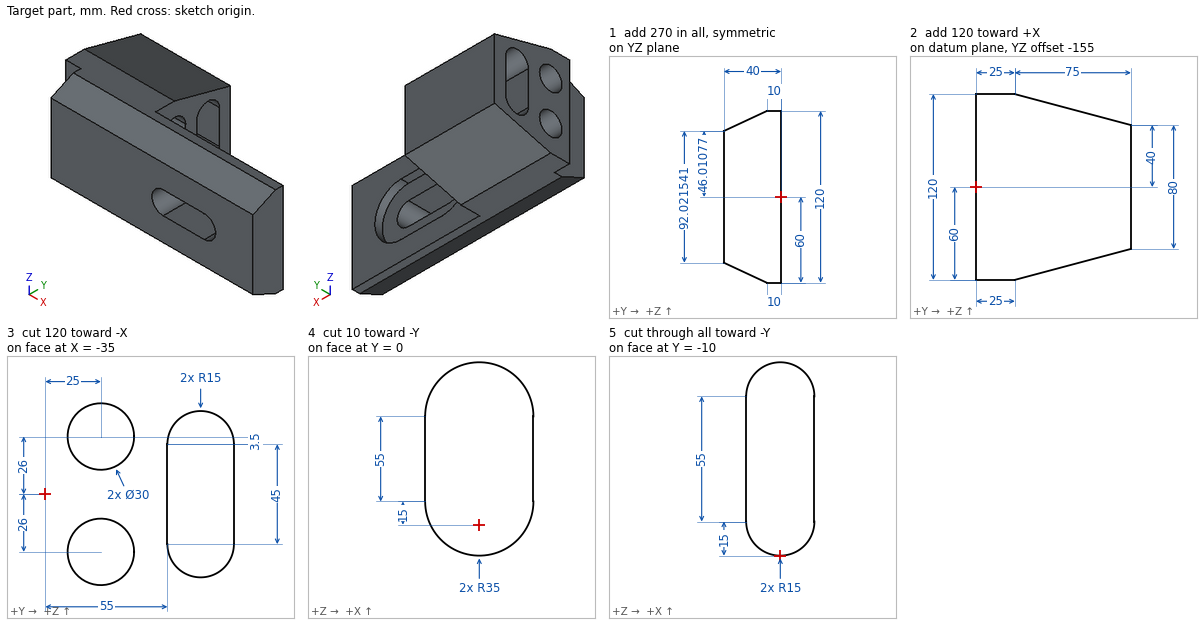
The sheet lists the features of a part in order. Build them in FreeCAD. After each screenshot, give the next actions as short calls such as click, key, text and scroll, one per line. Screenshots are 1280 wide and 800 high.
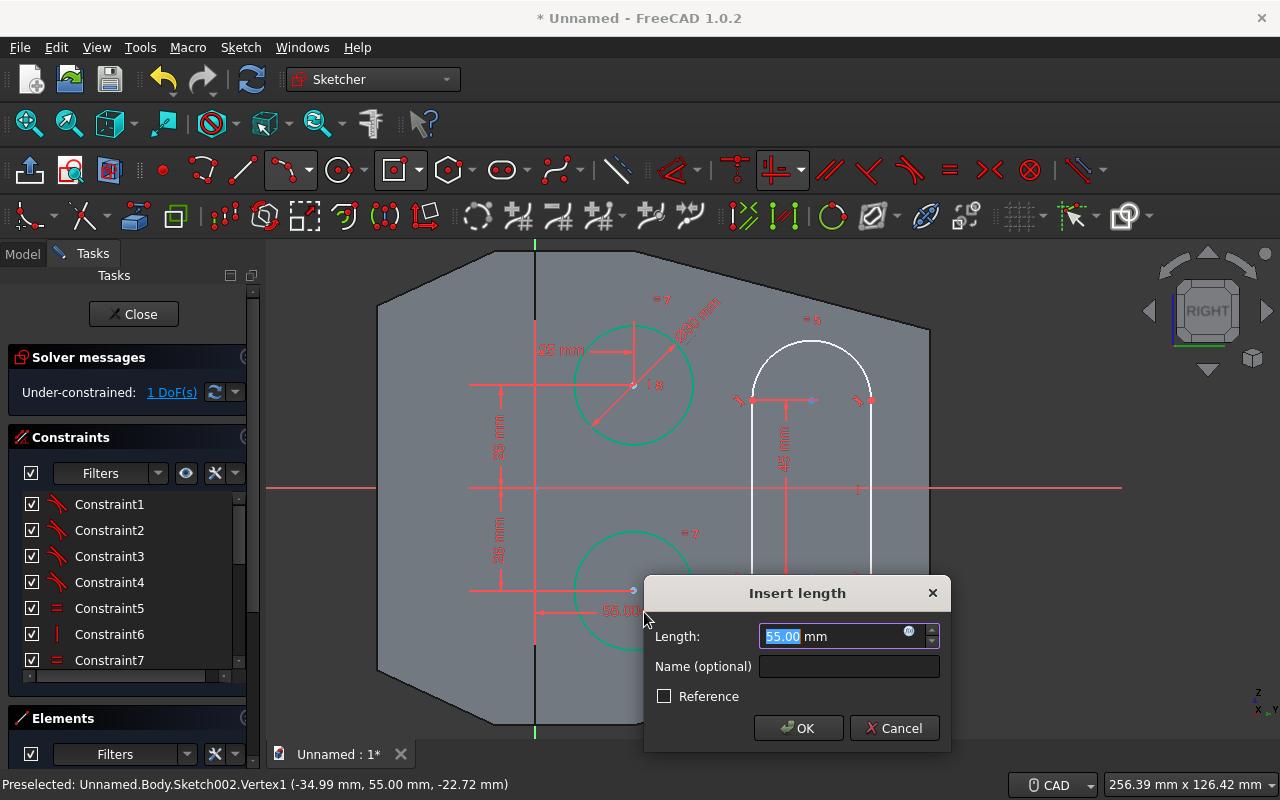
text(55)
key(Return)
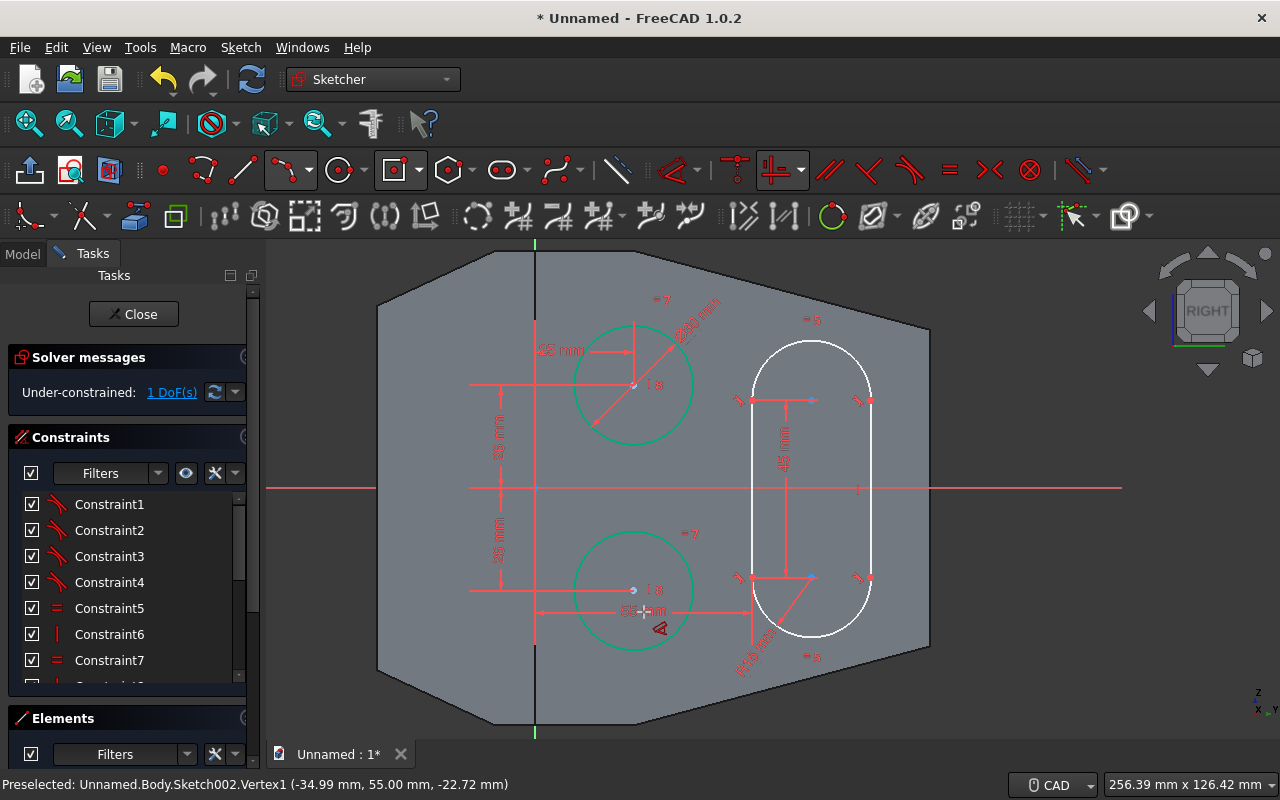
scroll(752, 400, up, 6)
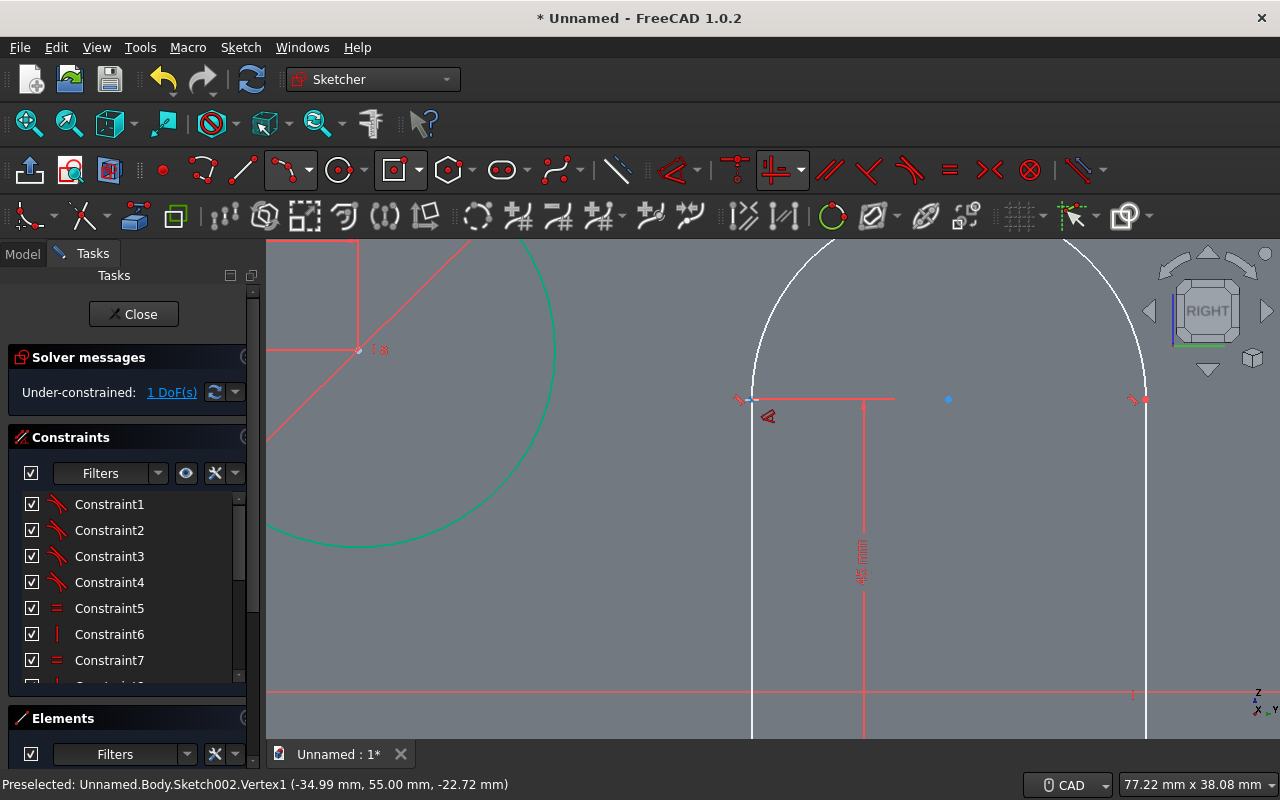
click(752, 399)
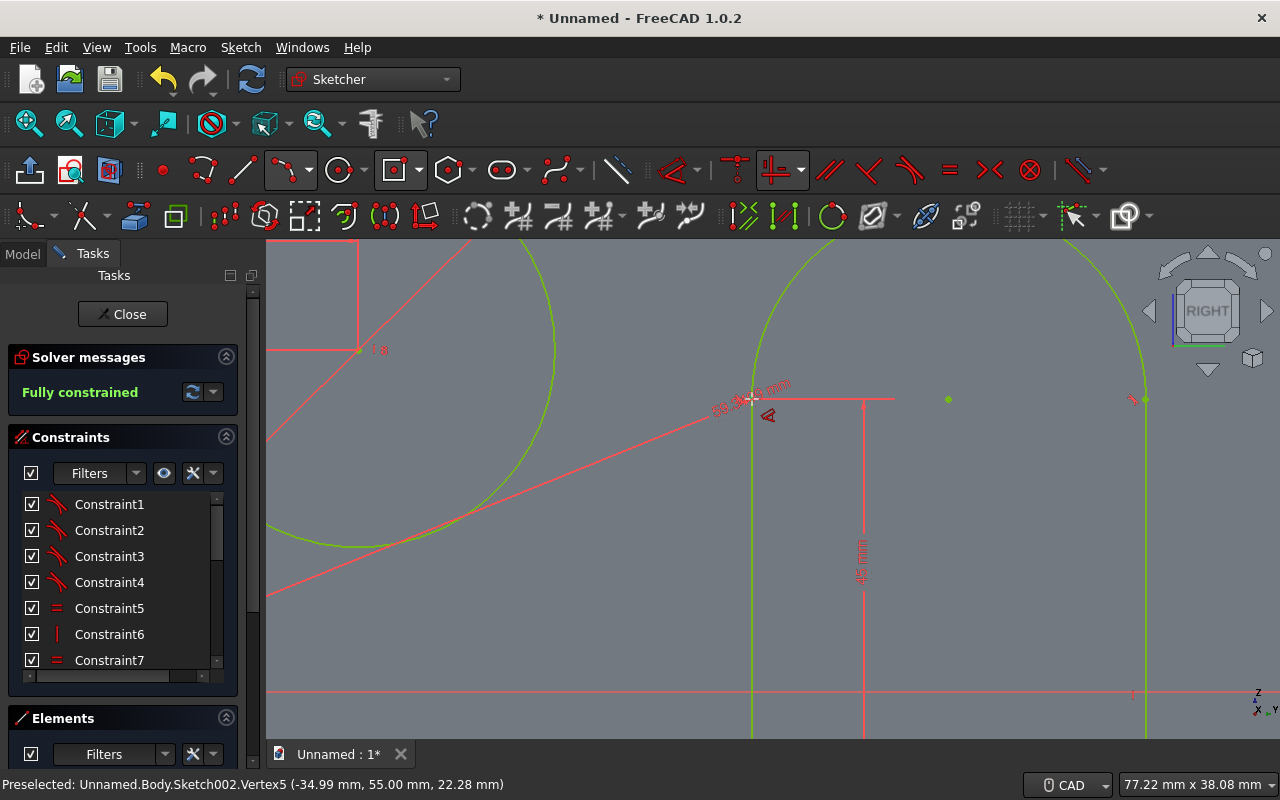
click(358, 350)
click(324, 375)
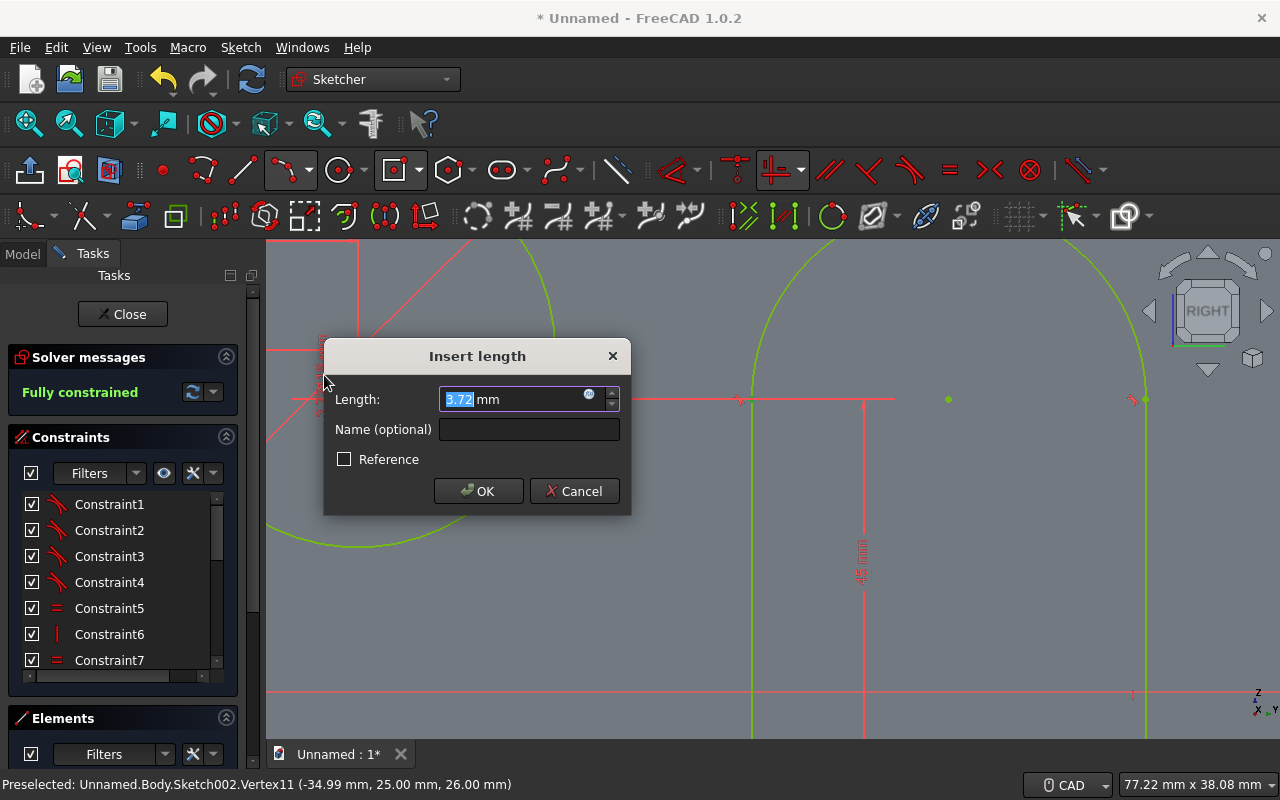
text(3.5)
key(Return)
key(Escape)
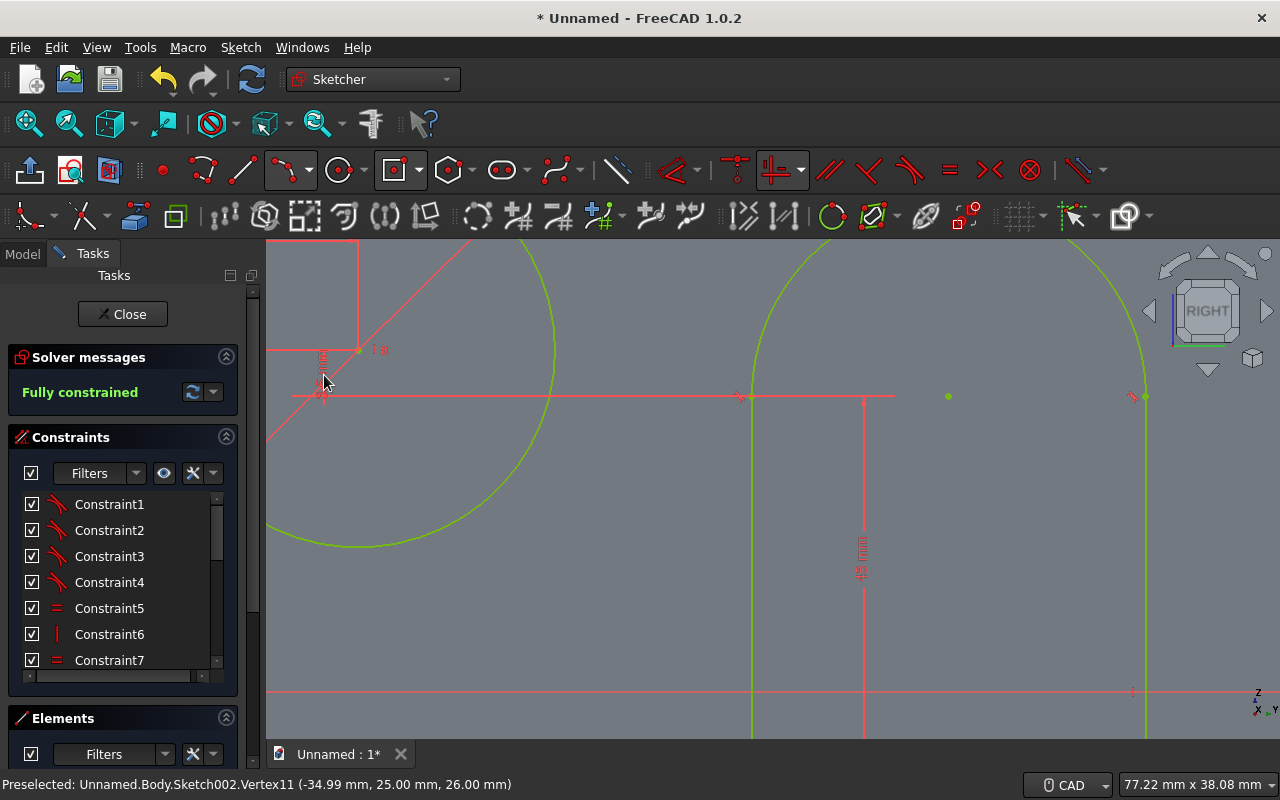
click(123, 314)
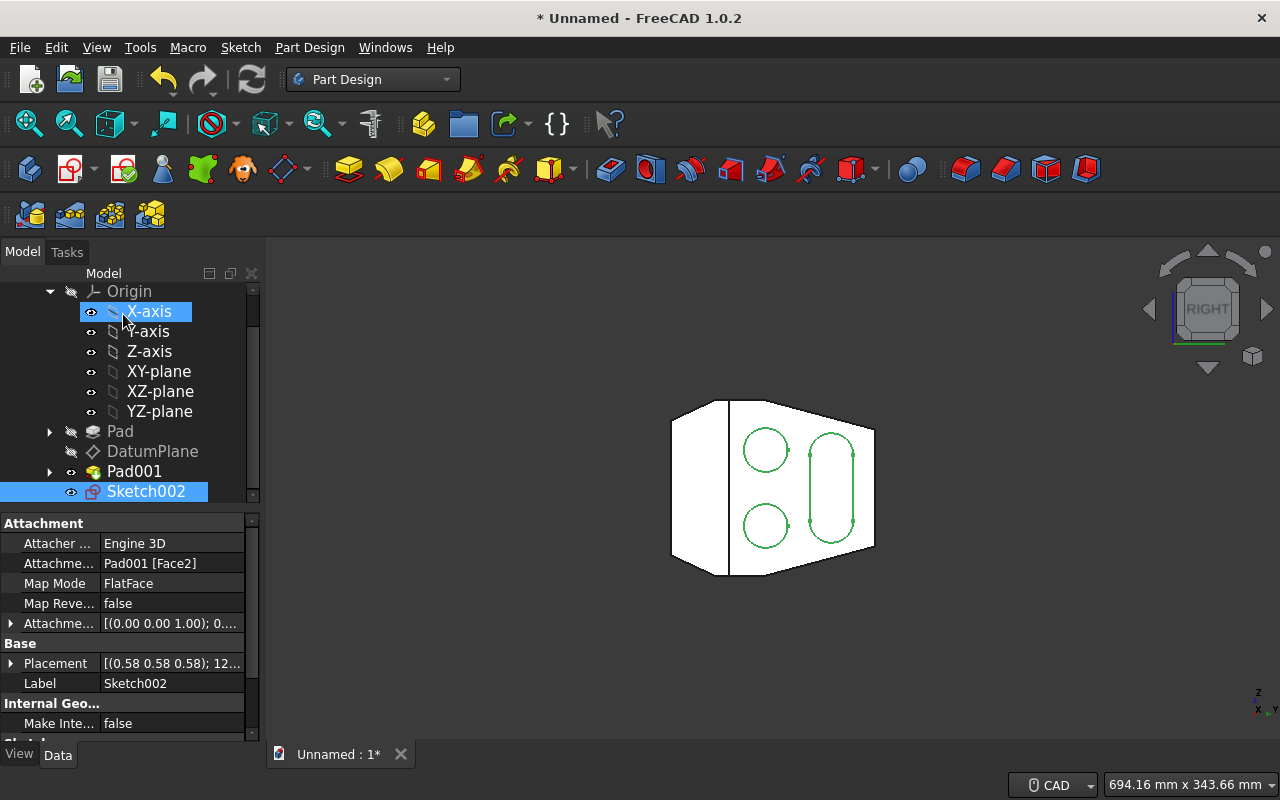
click(612, 170)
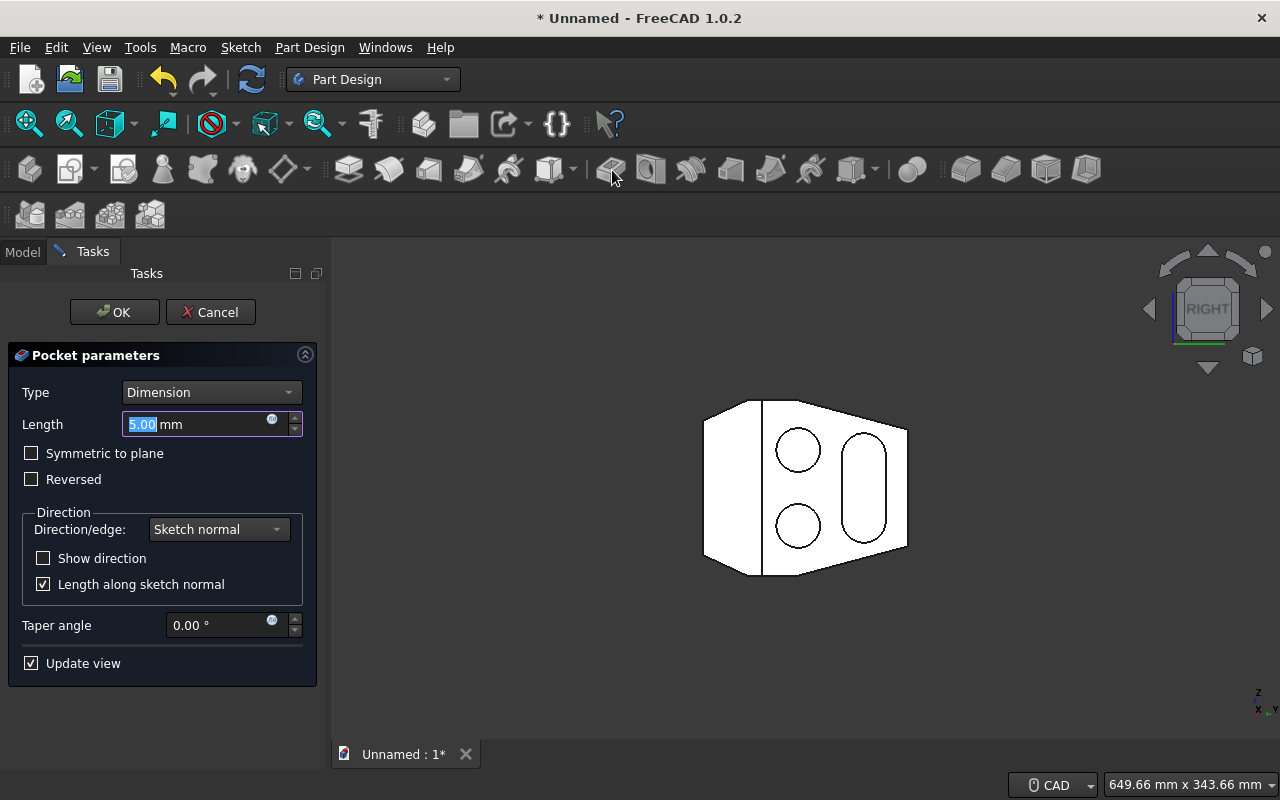
text(120)
key(Tab)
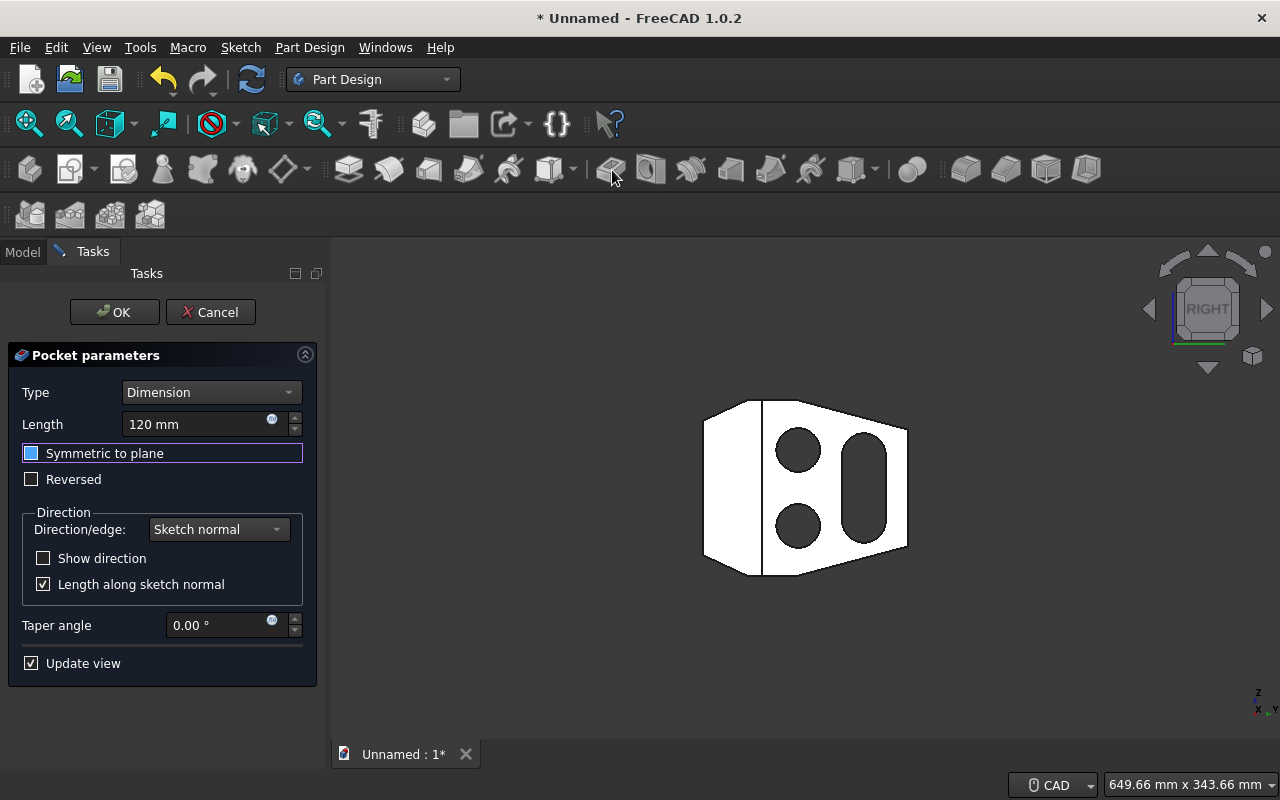
click(115, 312)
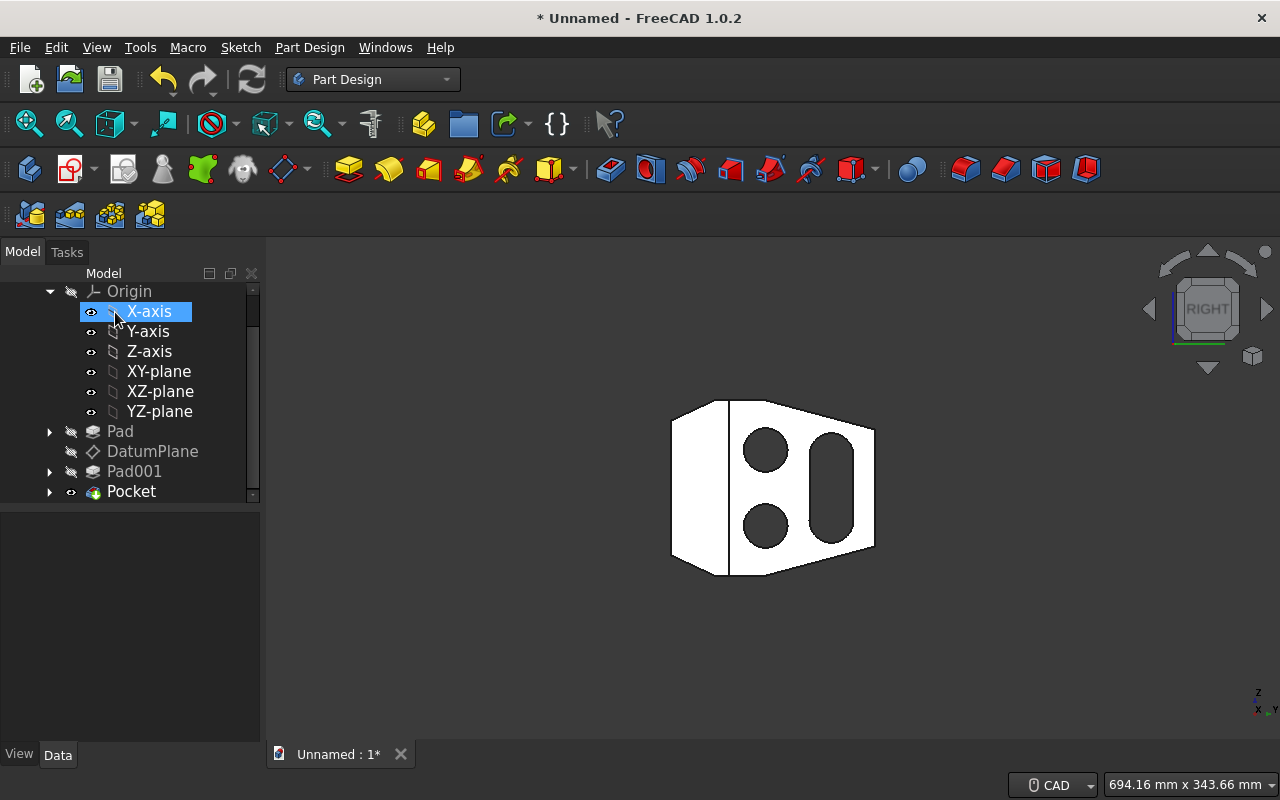
click(30, 124)